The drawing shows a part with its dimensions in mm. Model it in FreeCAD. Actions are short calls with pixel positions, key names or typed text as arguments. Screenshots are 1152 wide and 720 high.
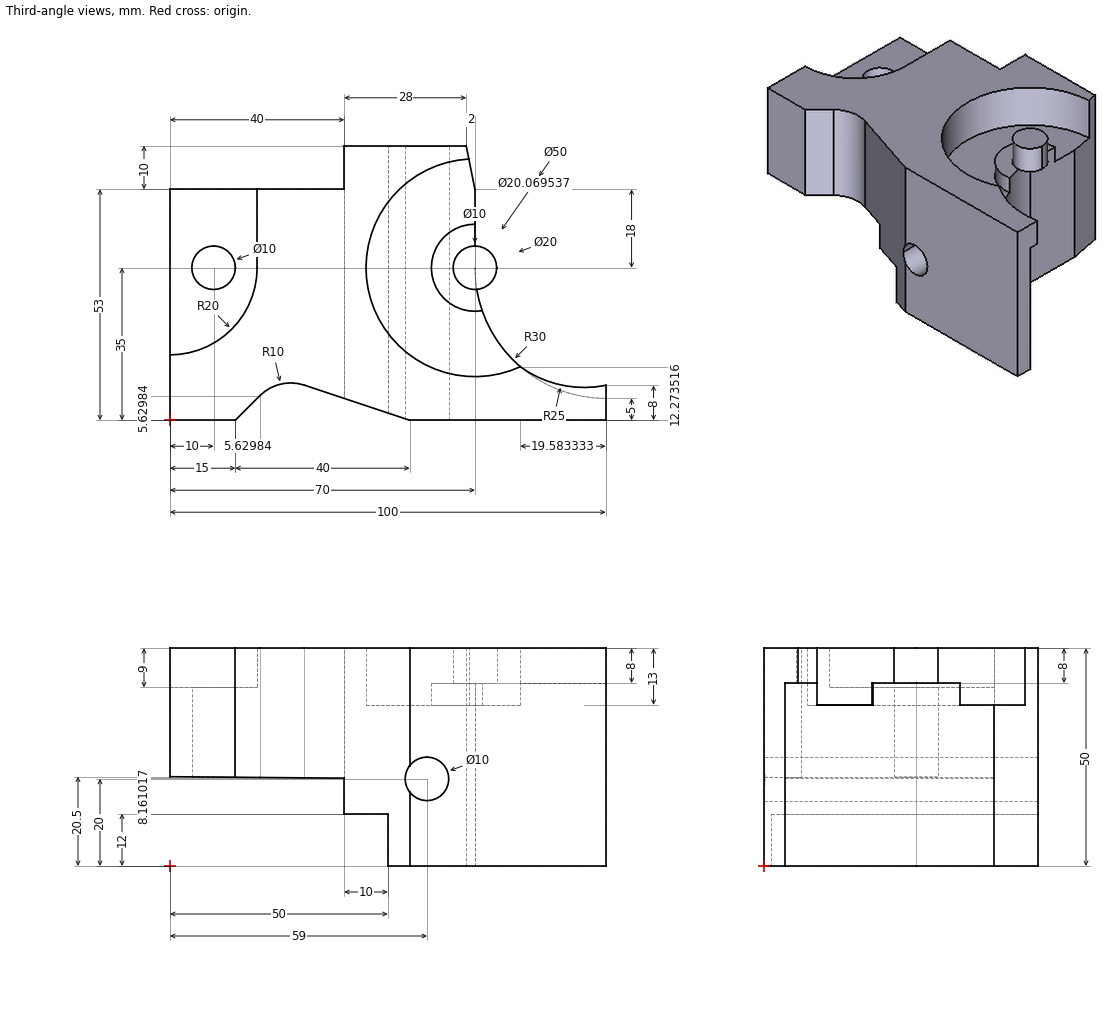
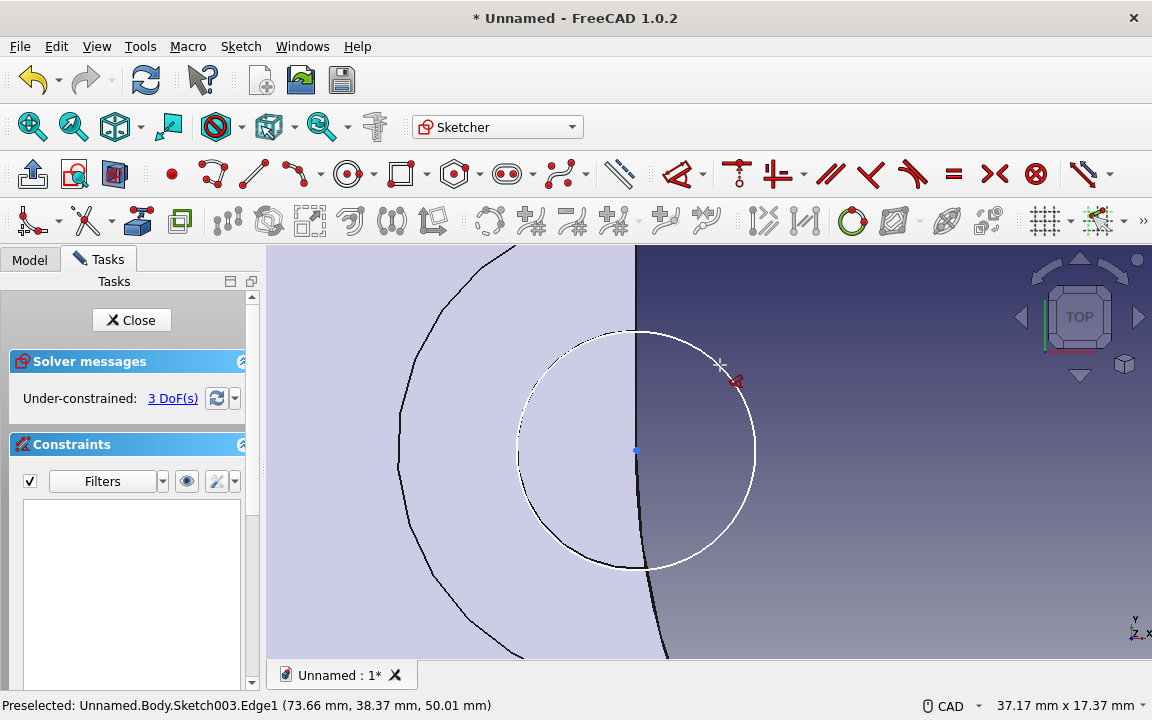
click(720, 366)
click(742, 343)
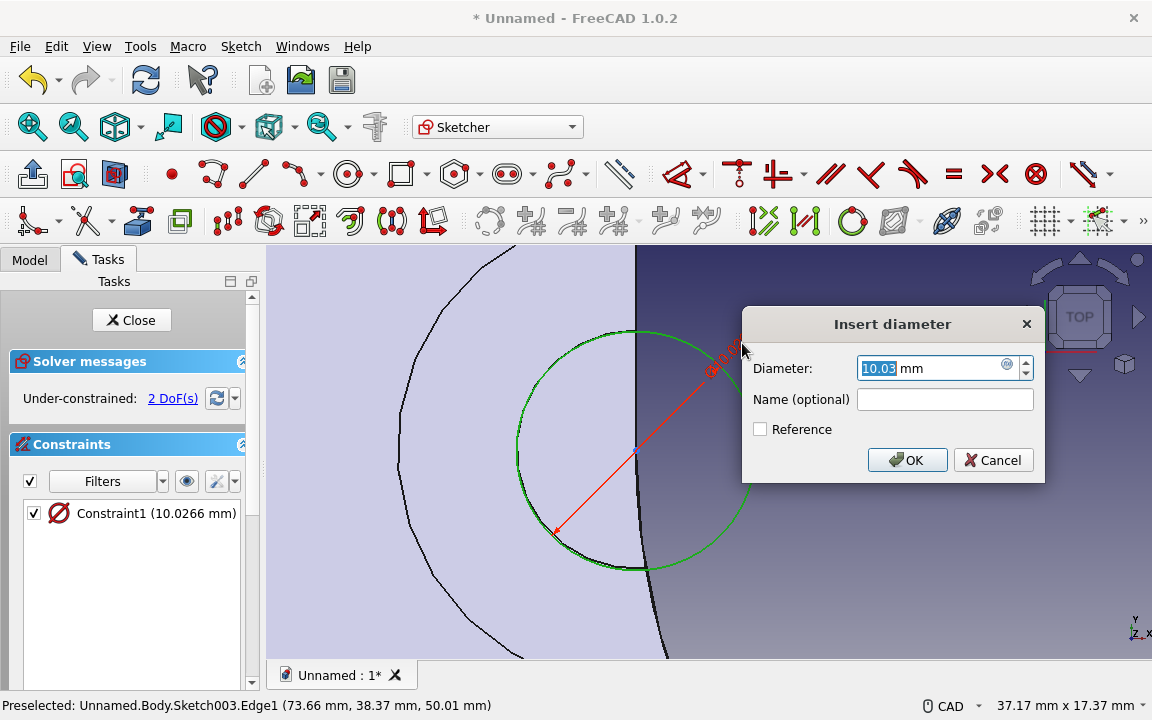
text(10)
key(Return)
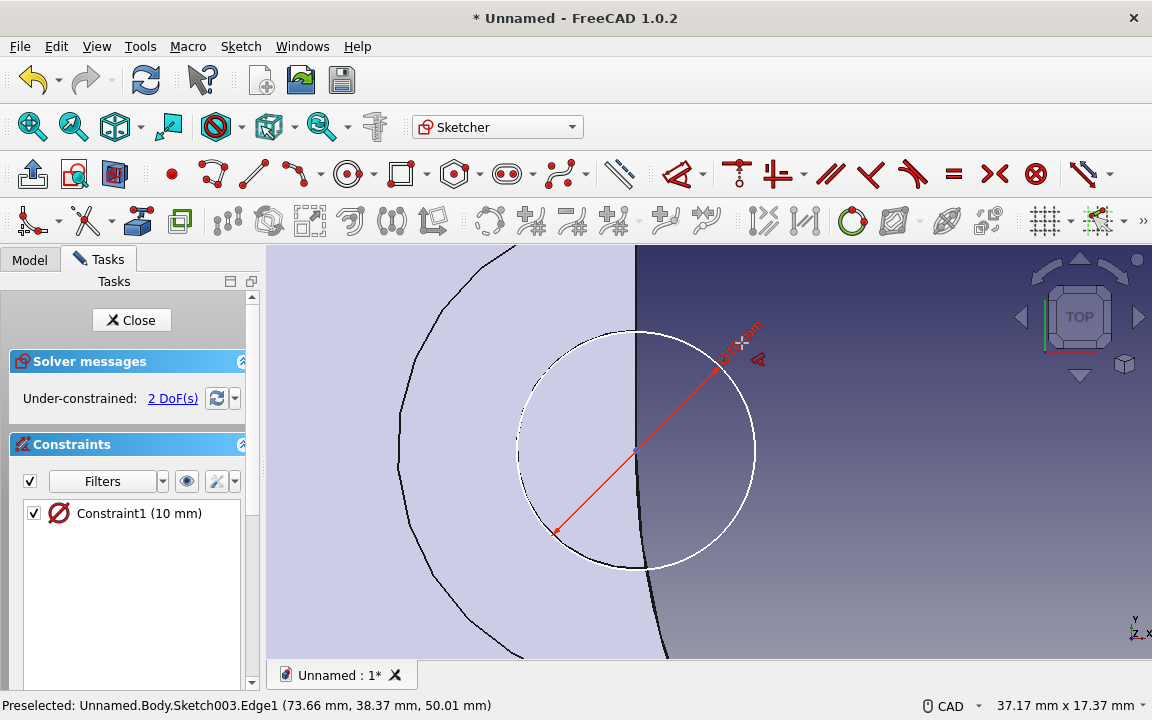
click(636, 451)
click(465, 417)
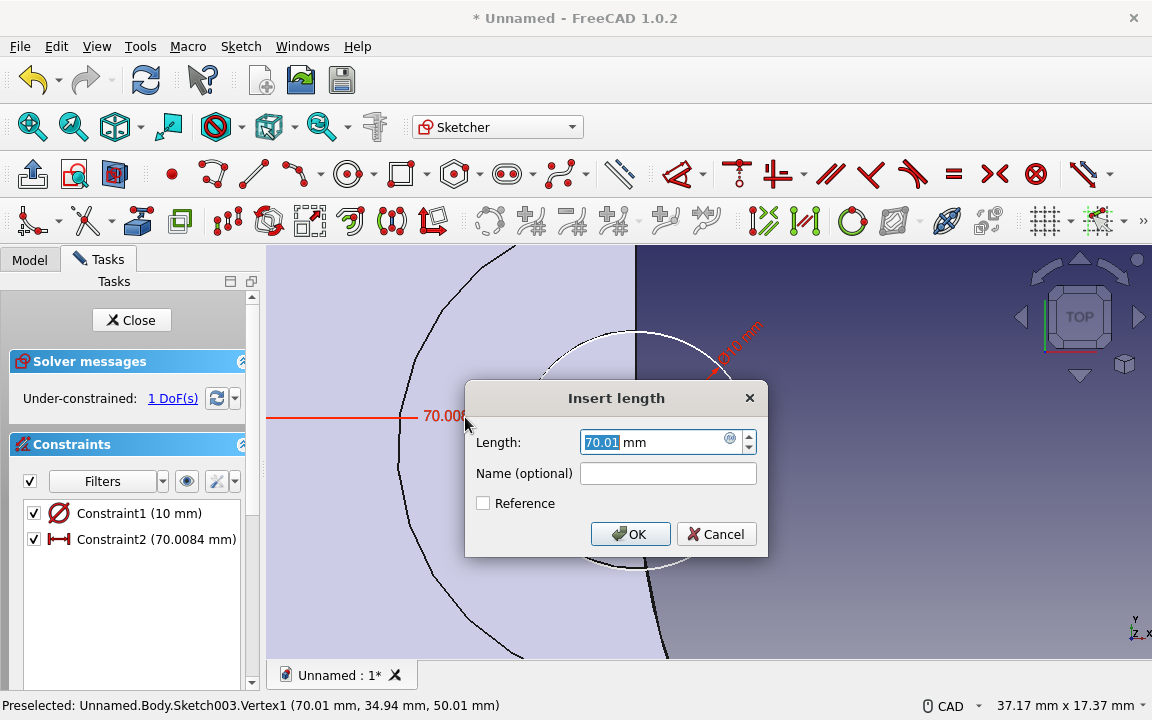
text(70)
key(Return)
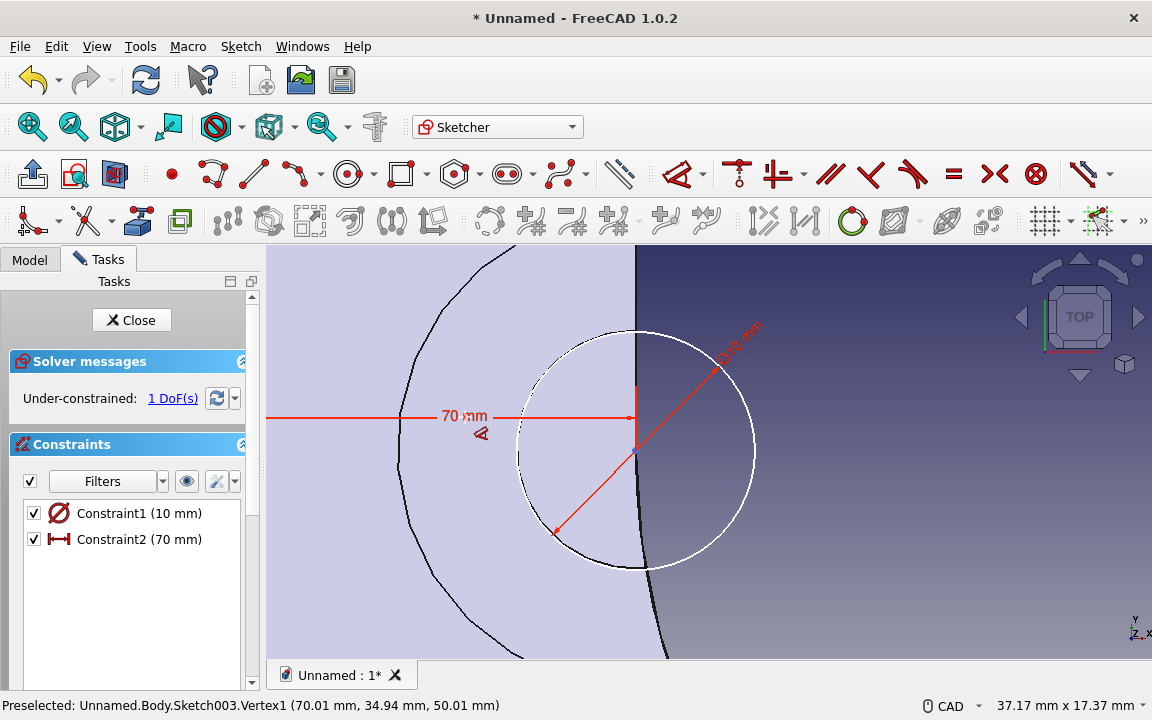
click(636, 451)
click(670, 541)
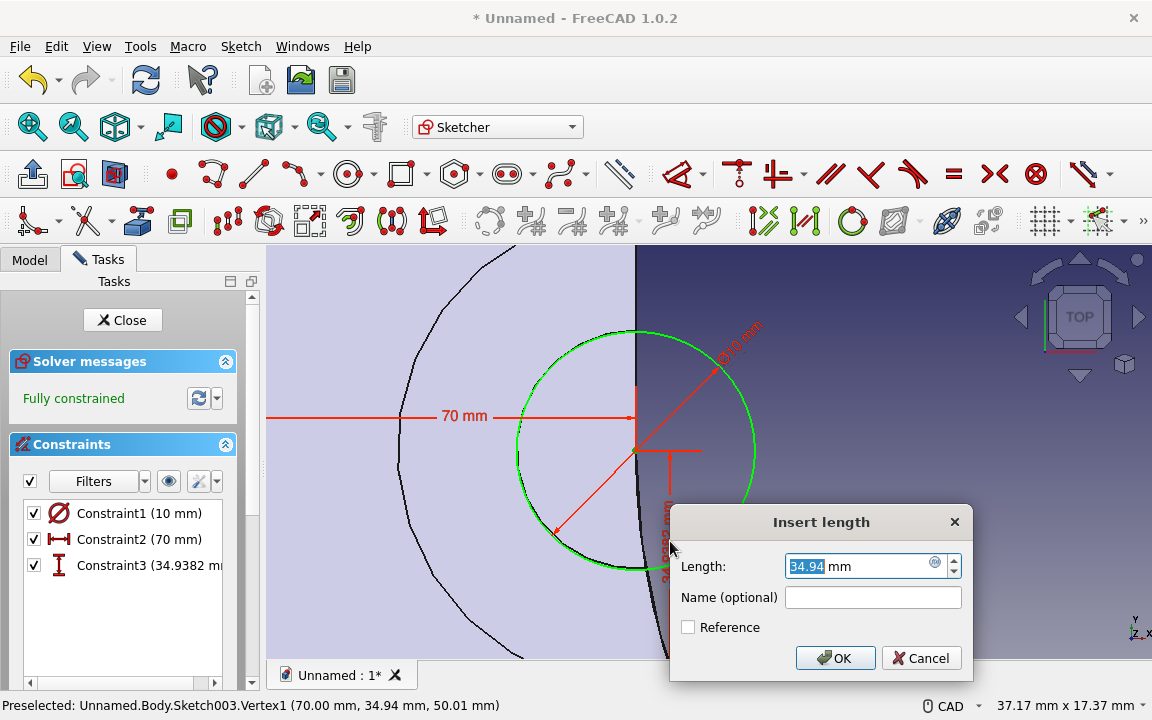
text(35)
key(Return)
key(Escape)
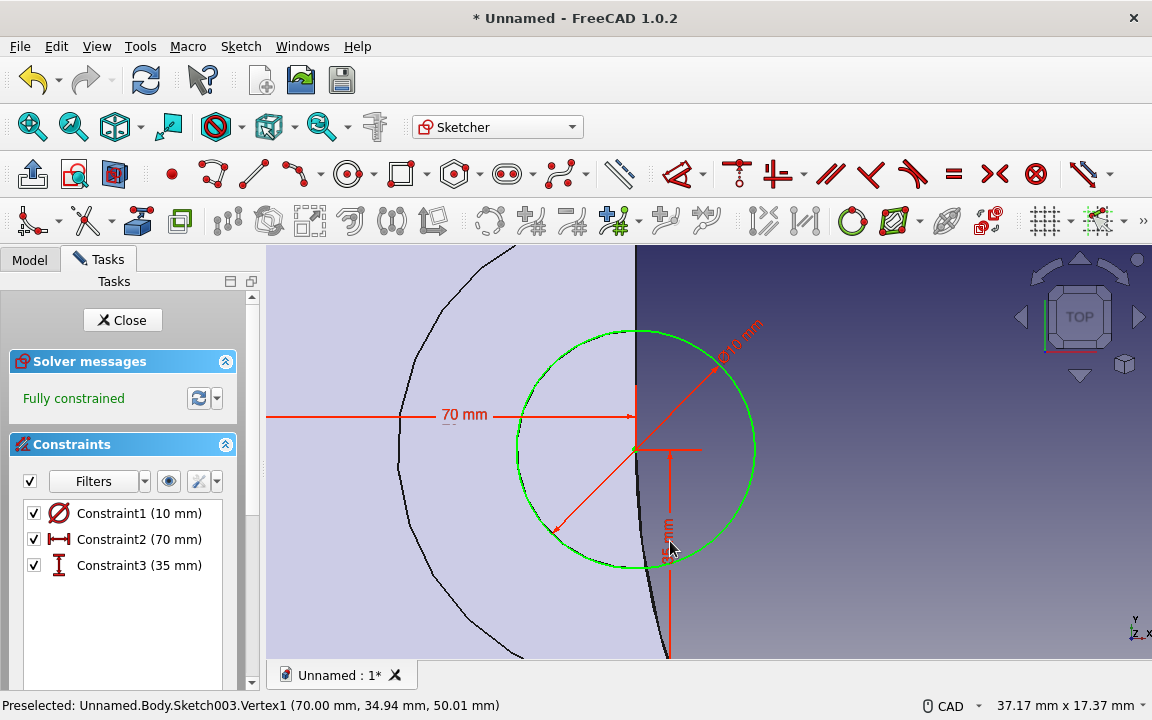
click(123, 320)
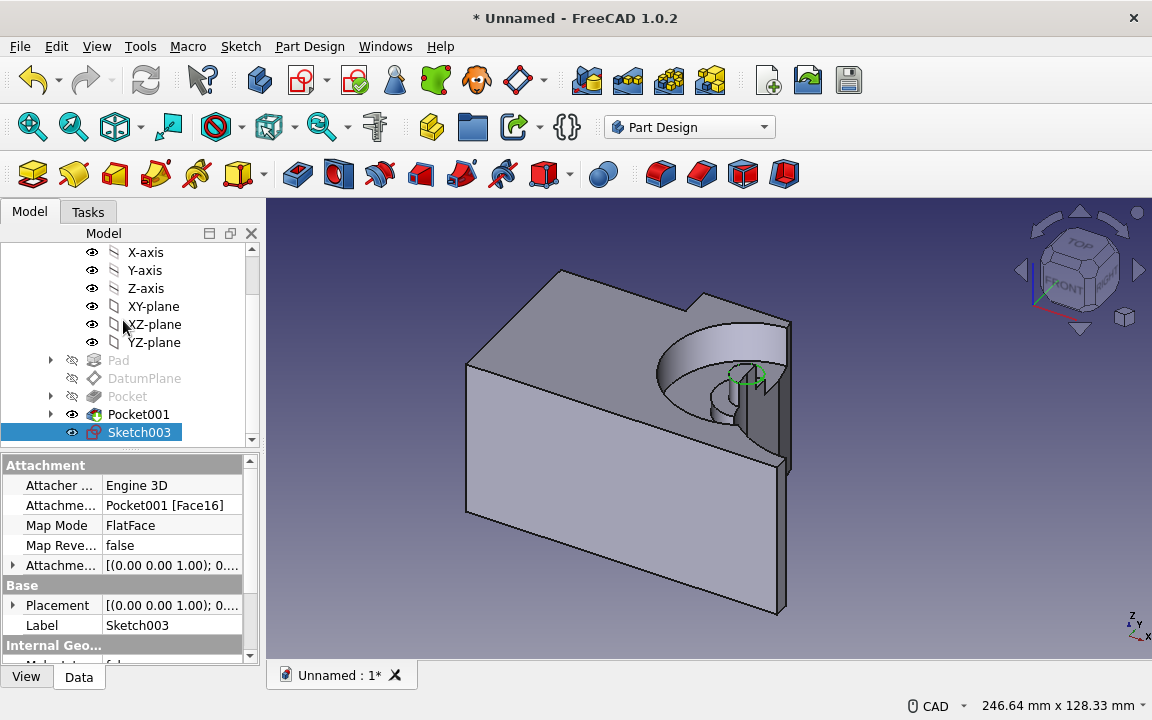
click(33, 174)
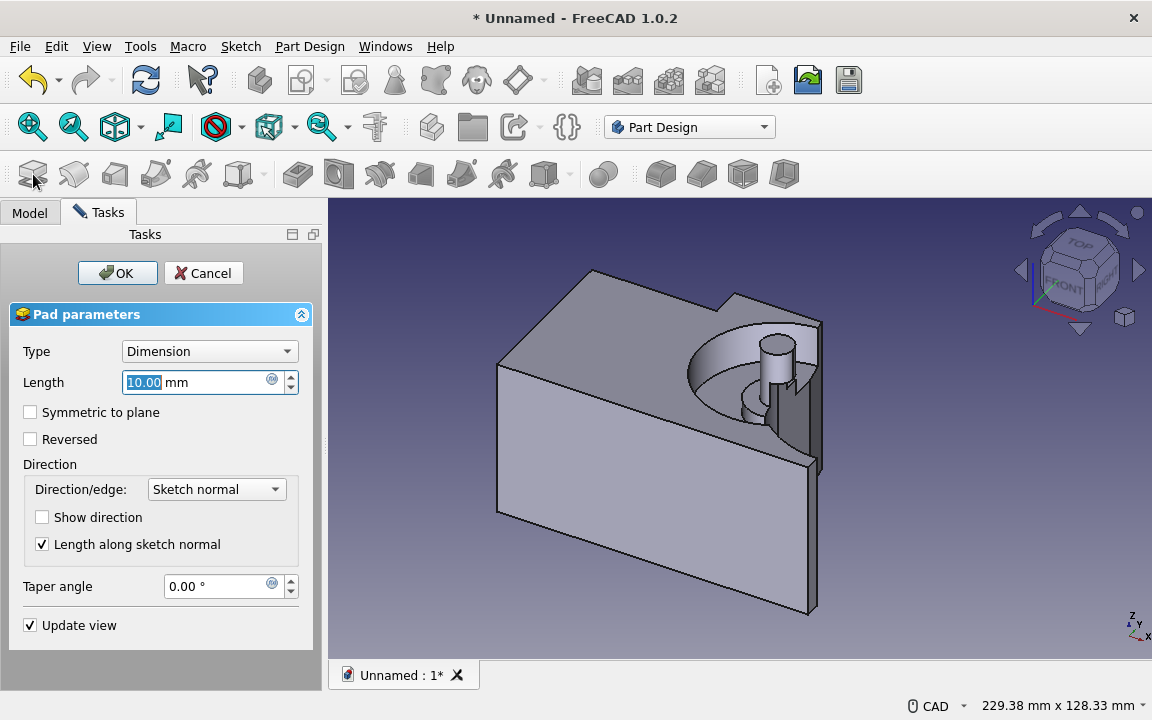
text(8)
key(Tab)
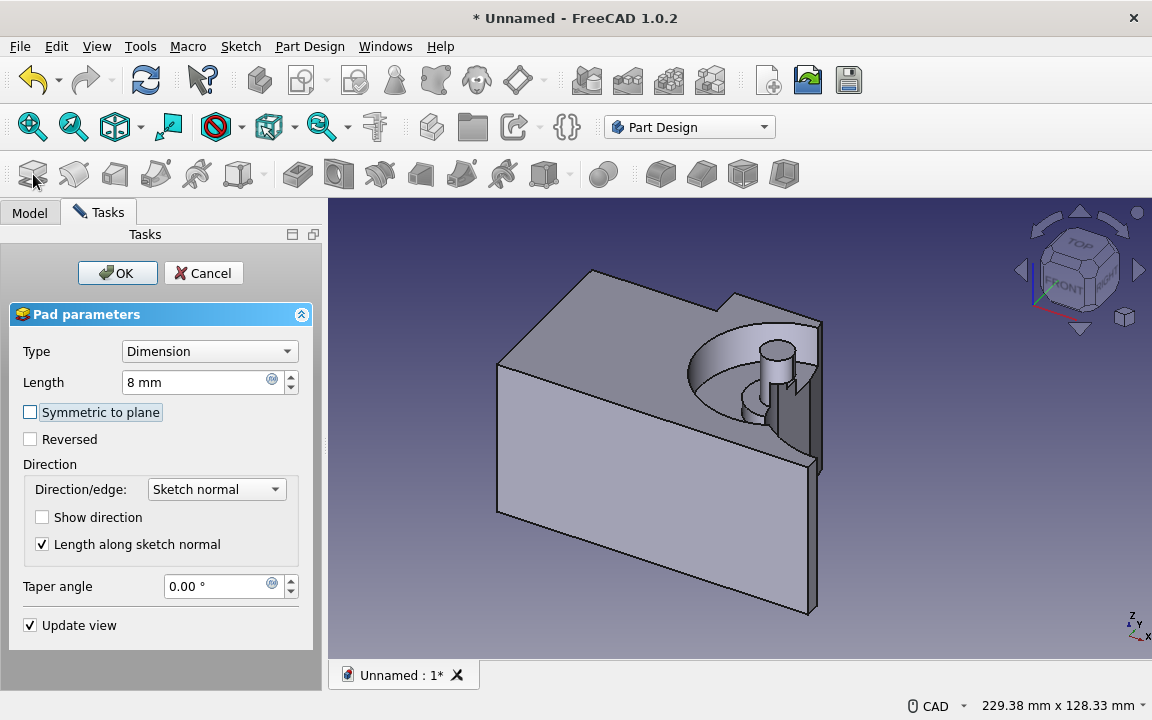
click(31, 439)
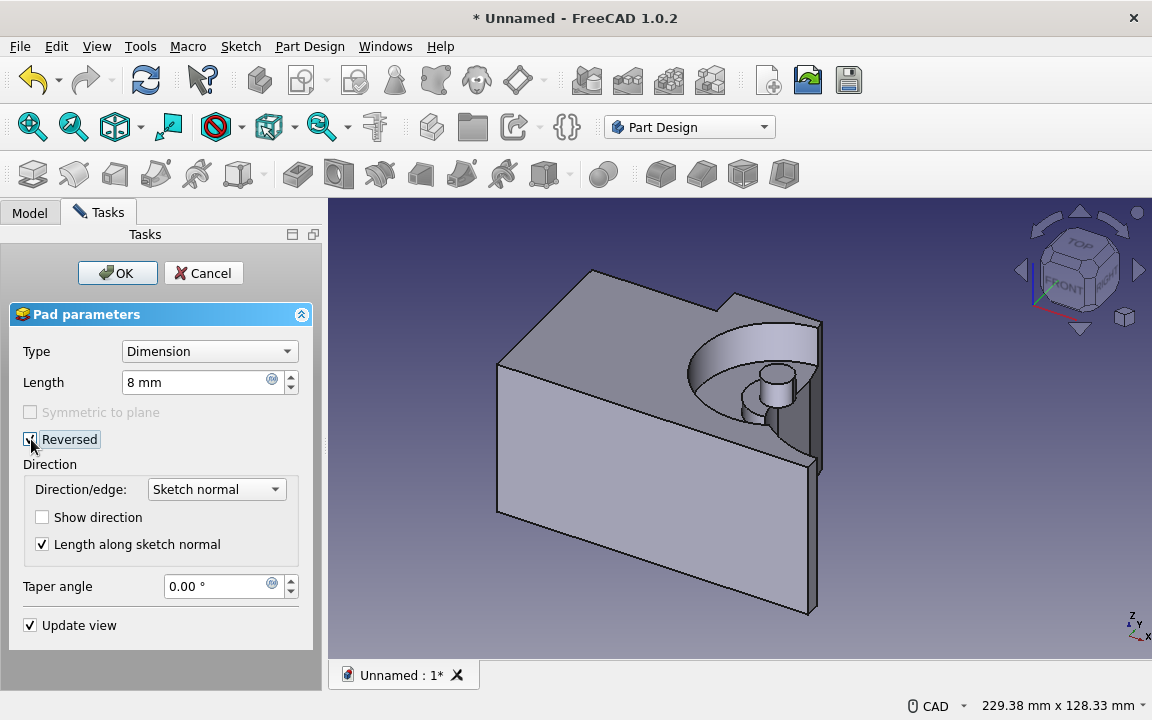
click(118, 273)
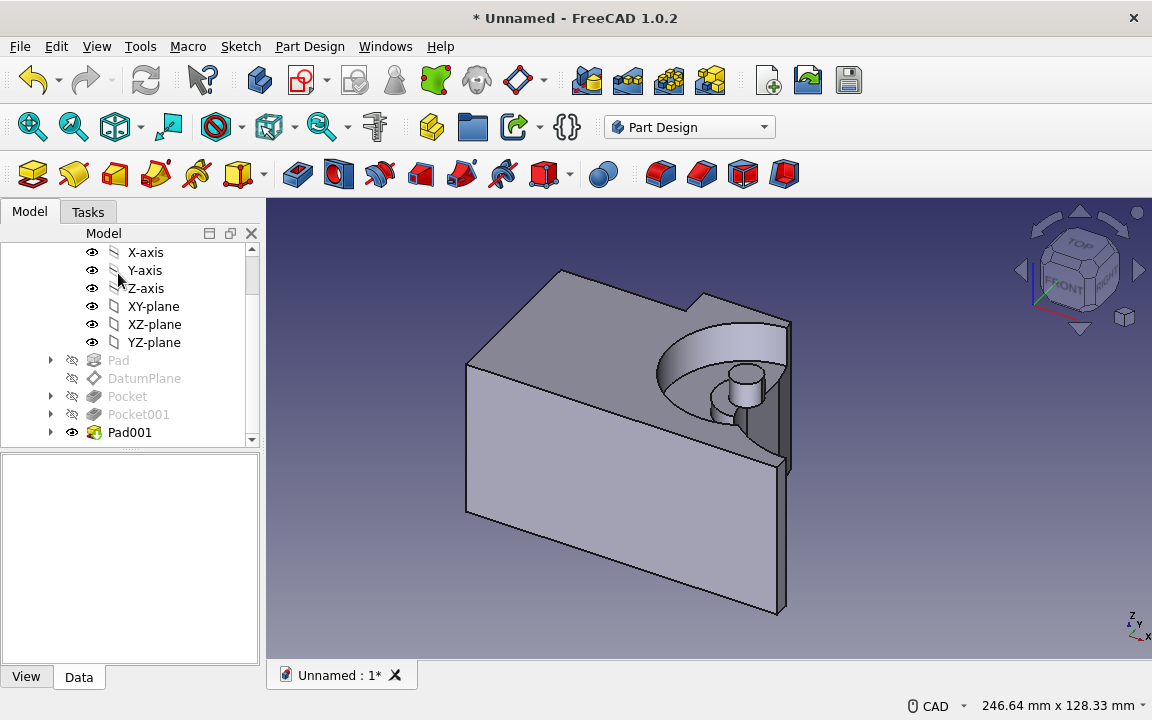
click(589, 329)